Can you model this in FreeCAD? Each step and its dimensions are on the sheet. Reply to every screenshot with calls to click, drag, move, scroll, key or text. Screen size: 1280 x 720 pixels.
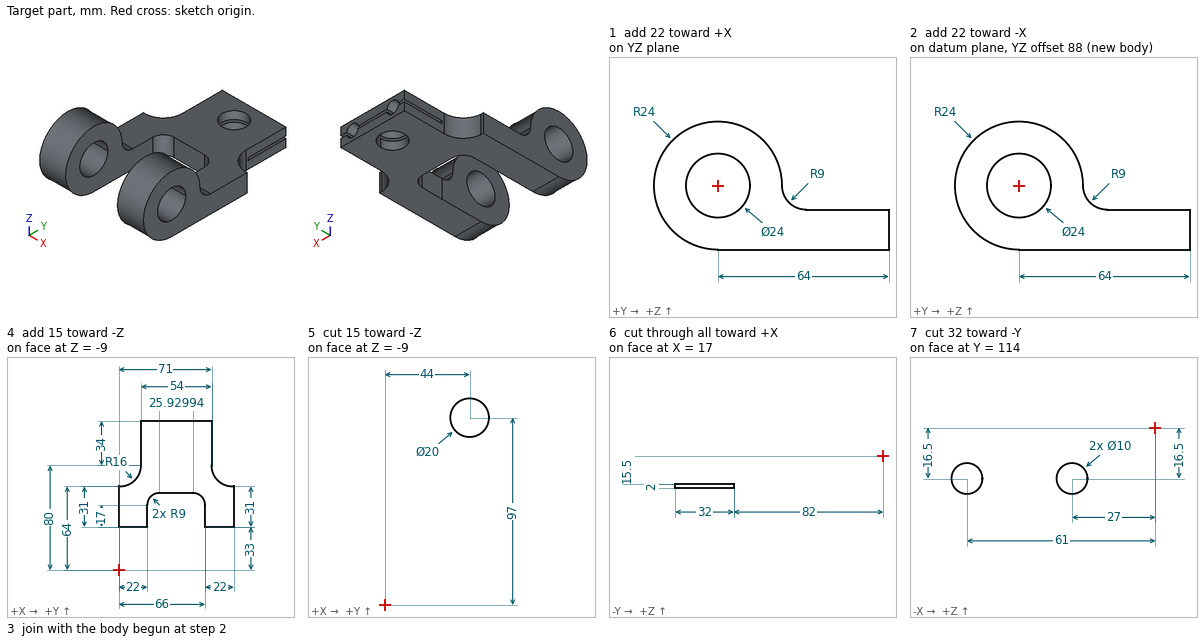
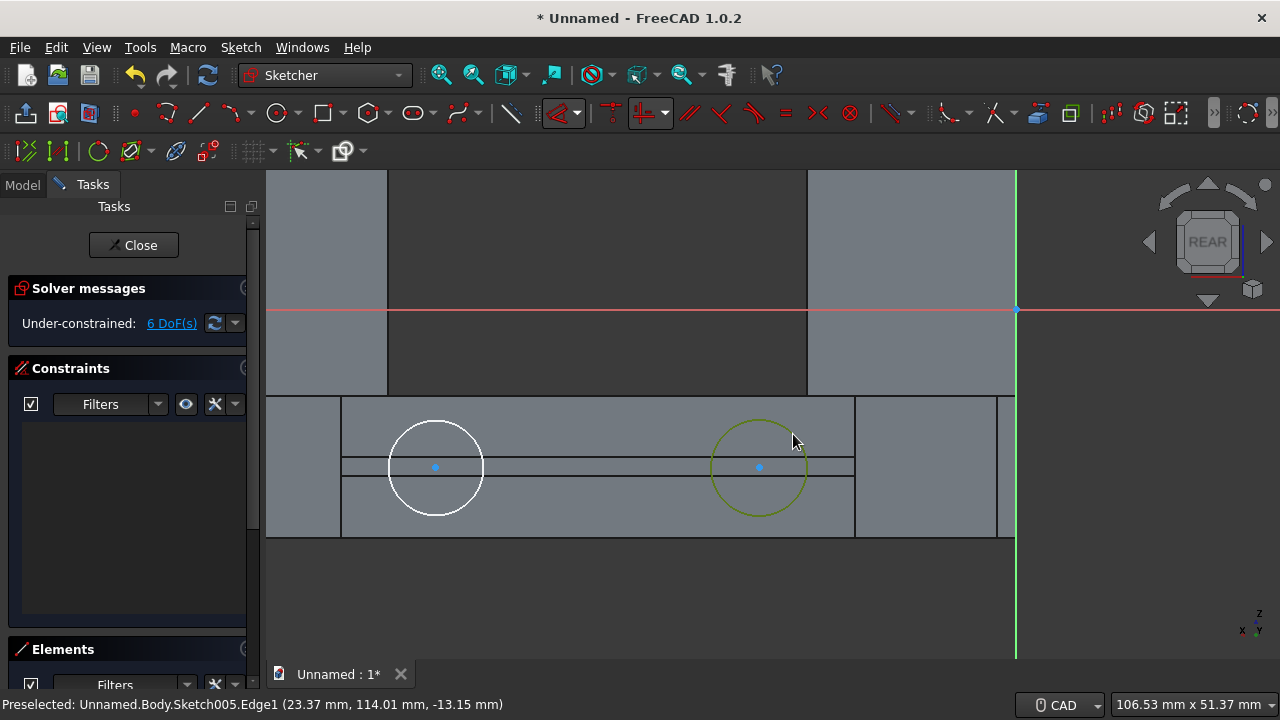
click(469, 434)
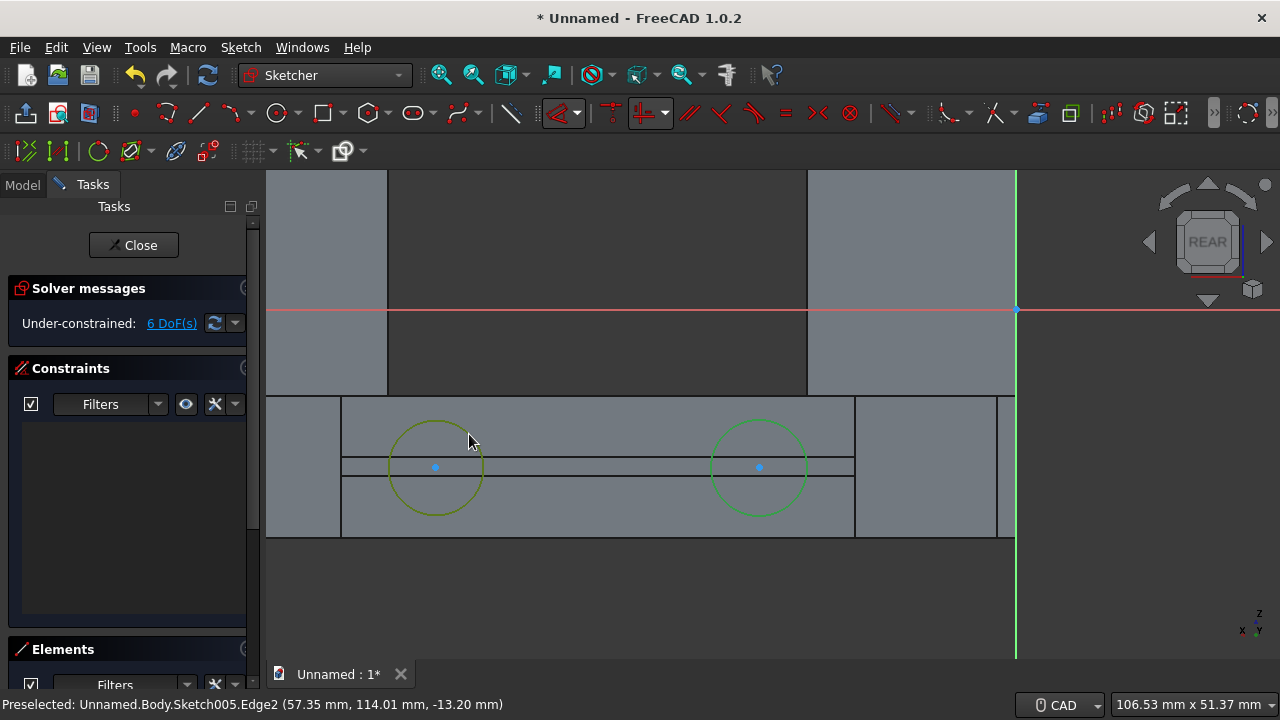
click(786, 114)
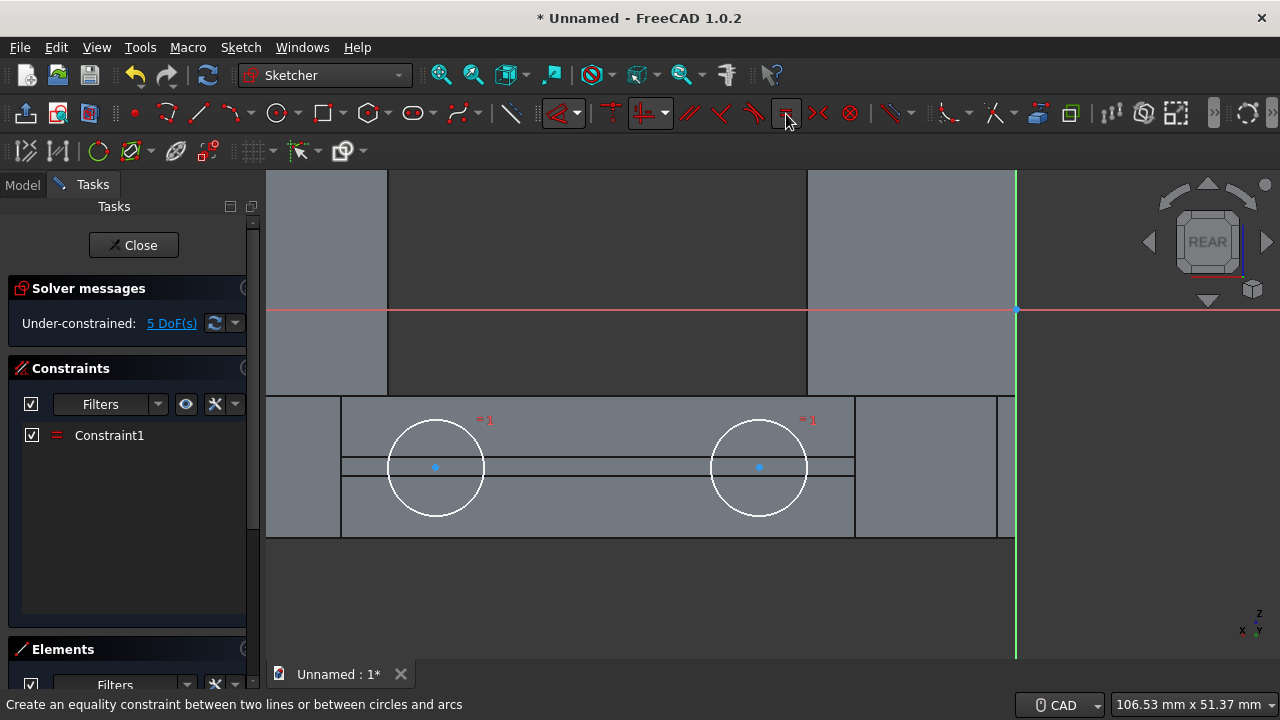
click(793, 434)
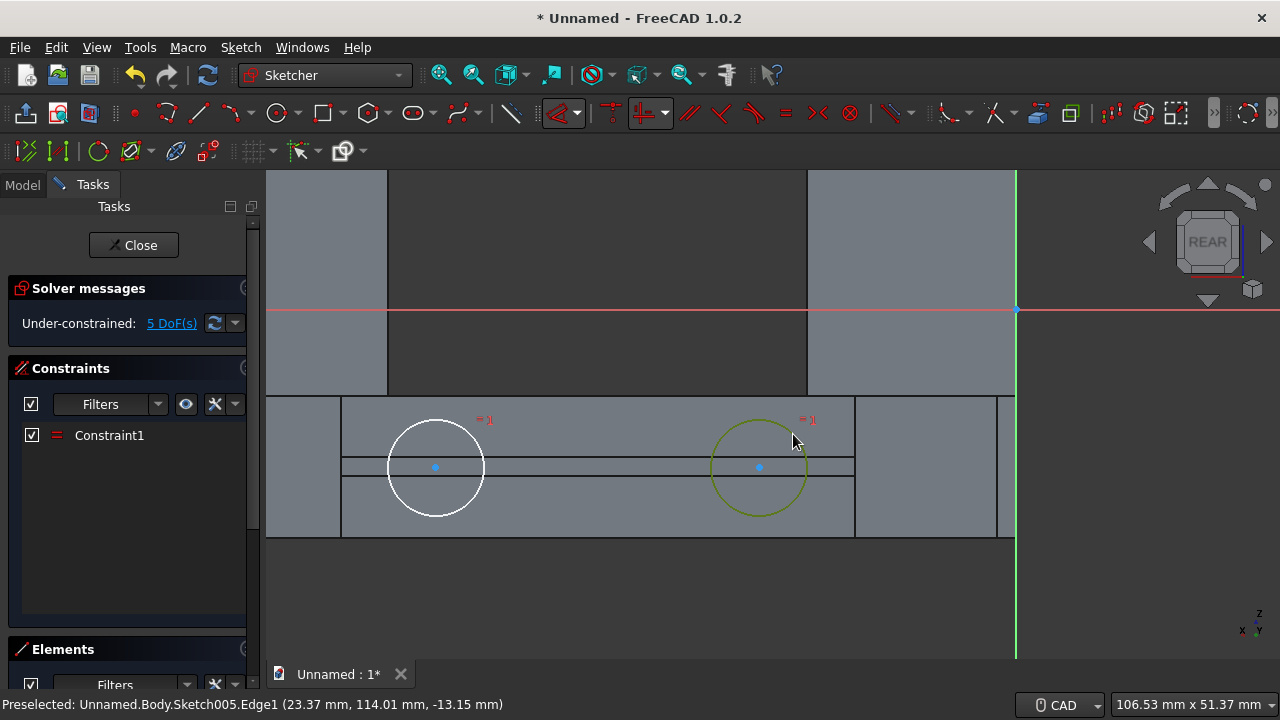
click(580, 114)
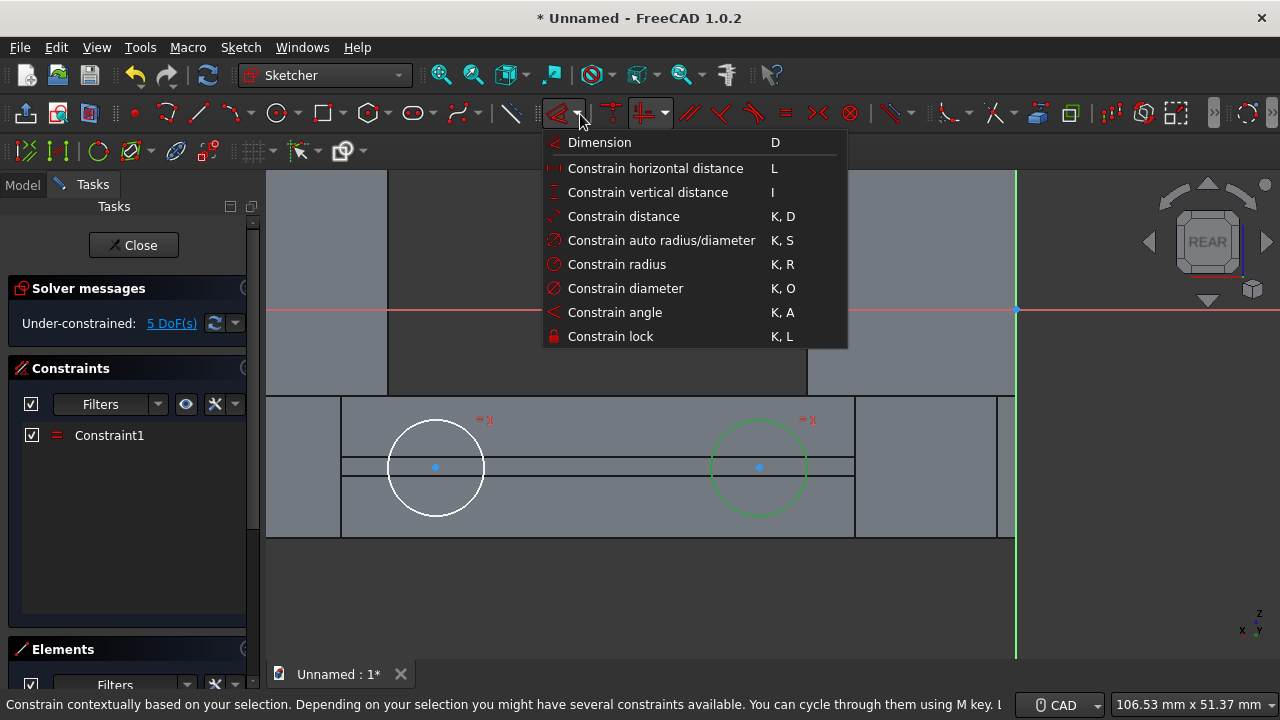
click(695, 288)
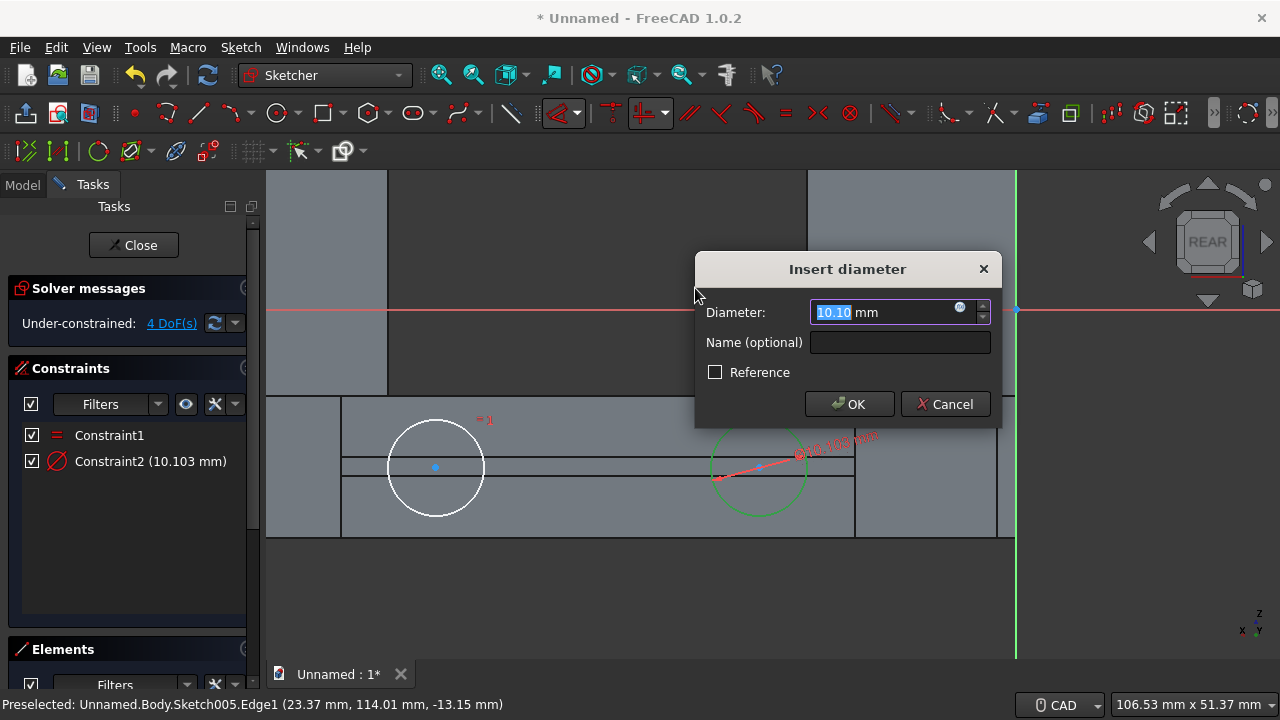
text(10)
key(Return)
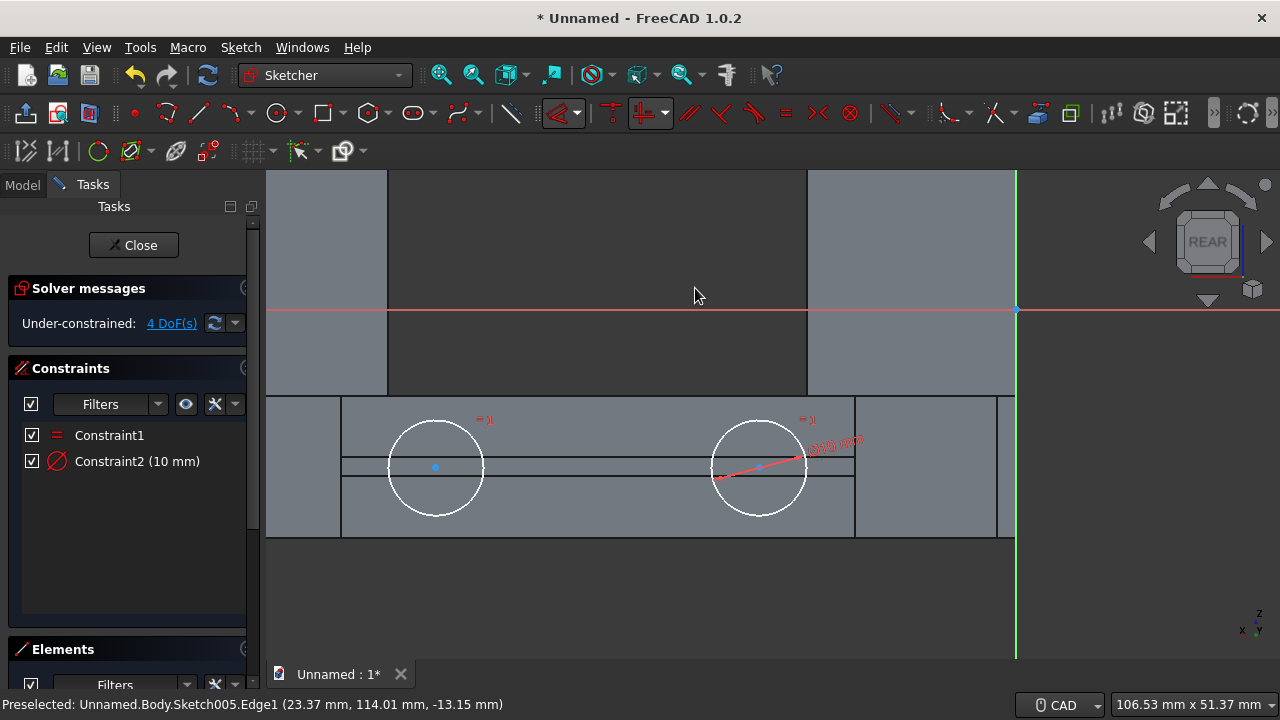
click(759, 468)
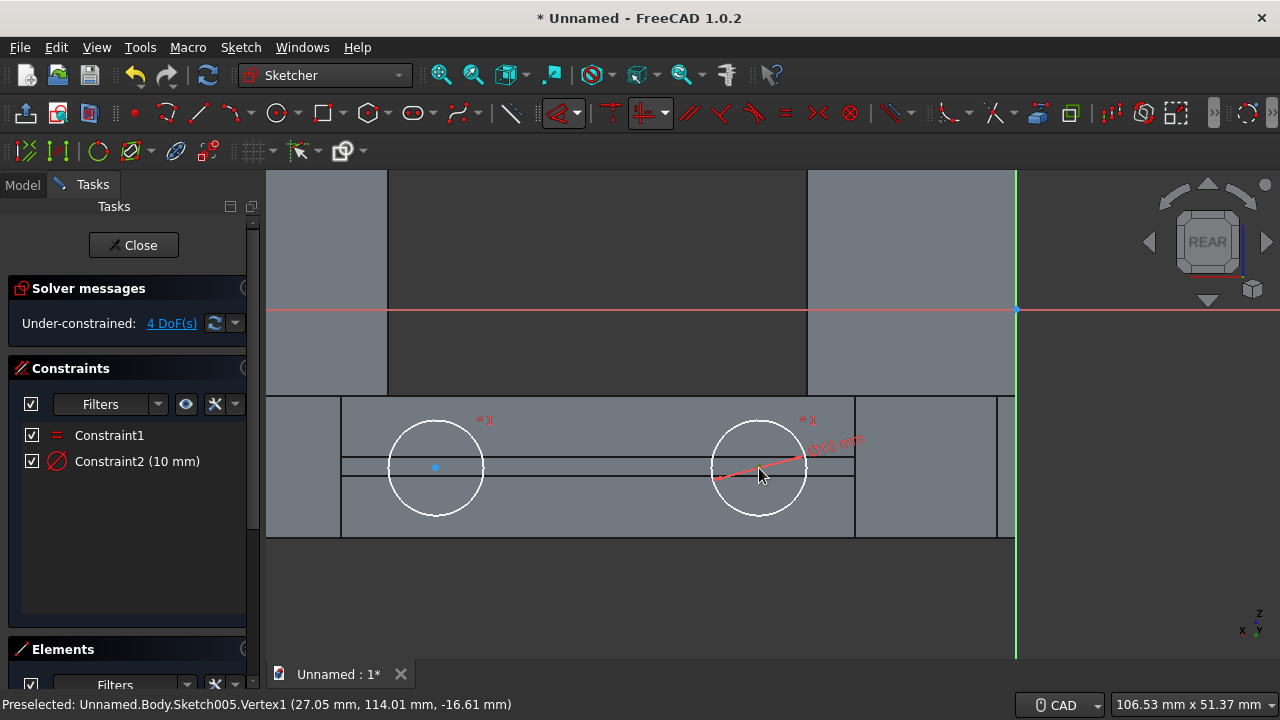
key(l)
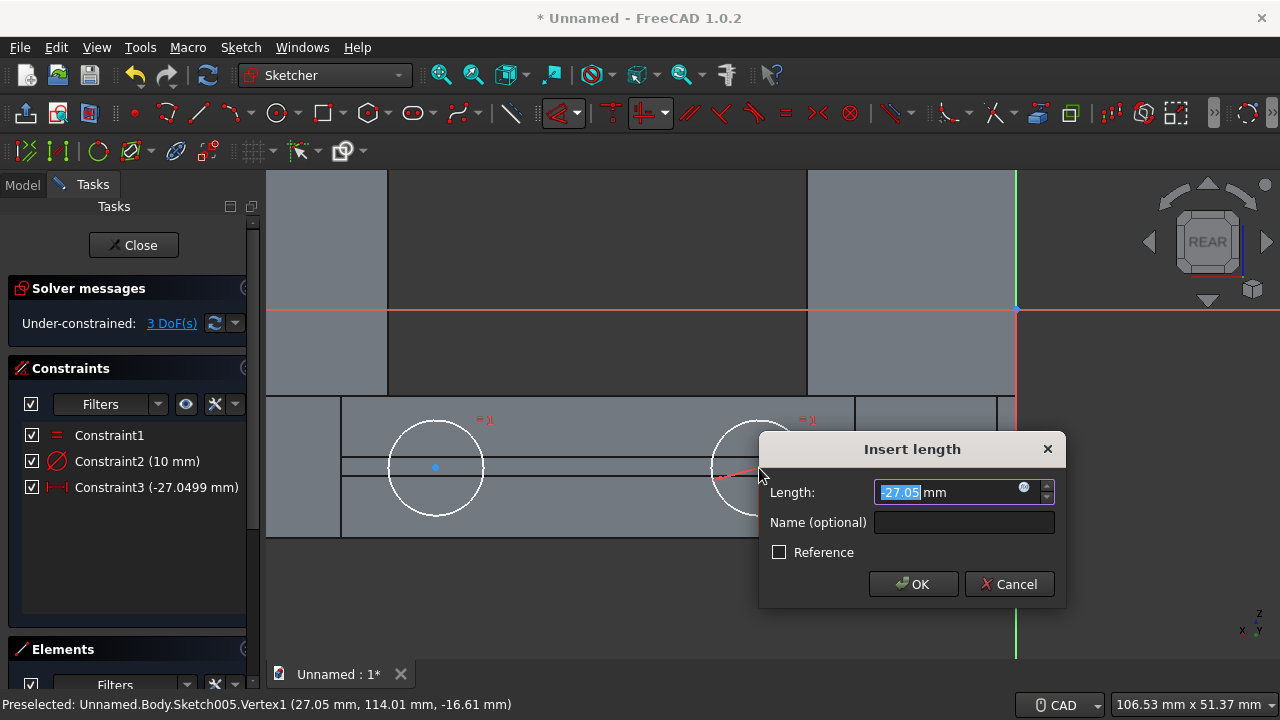
text(-27)
key(Return)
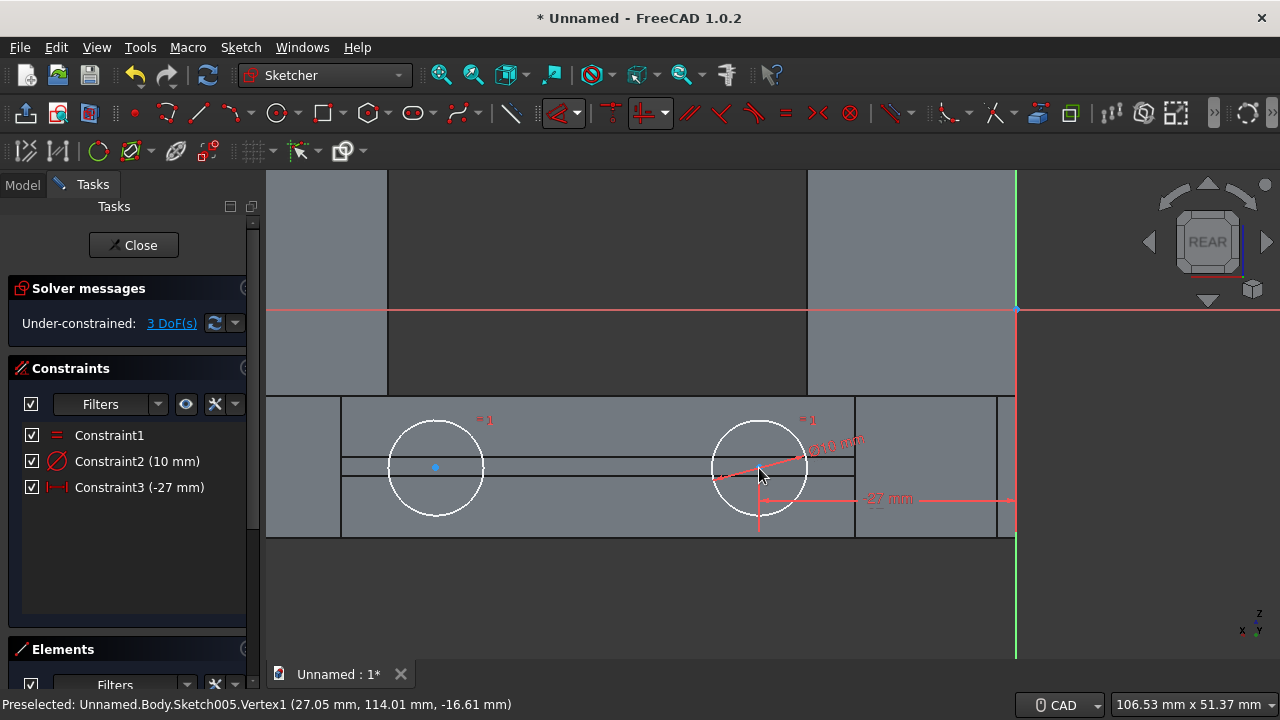
click(436, 468)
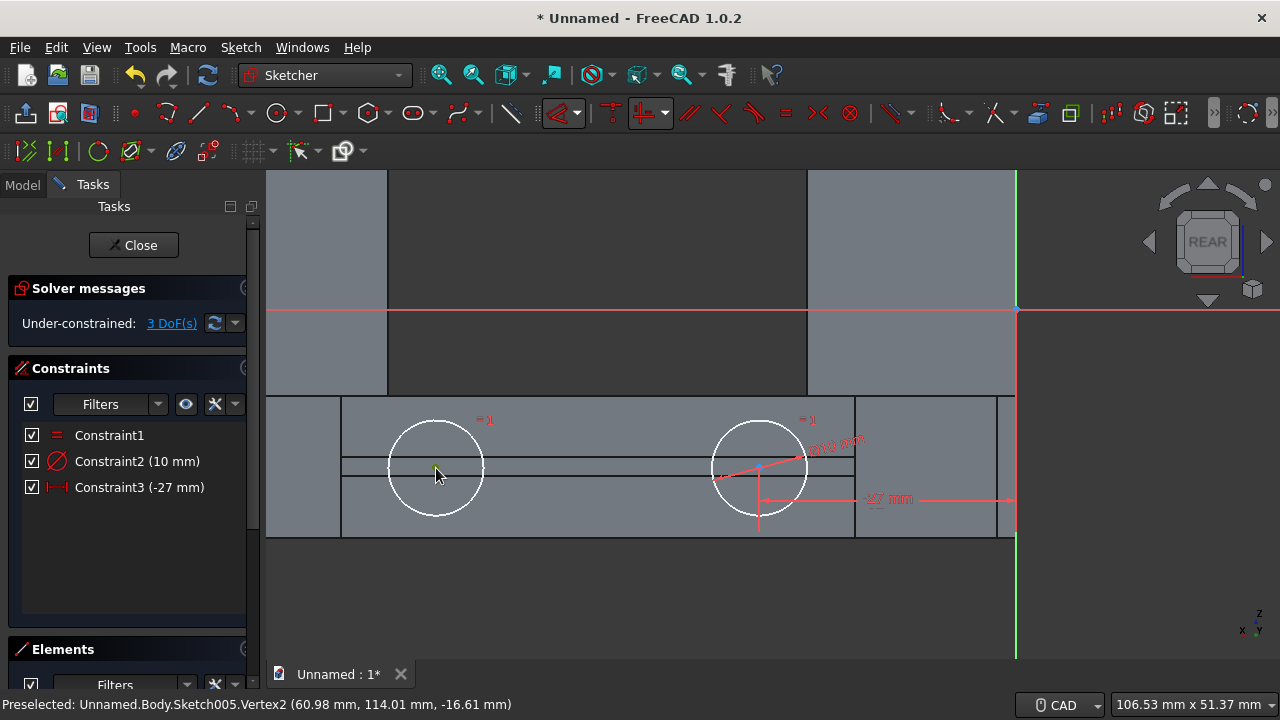
click(580, 114)